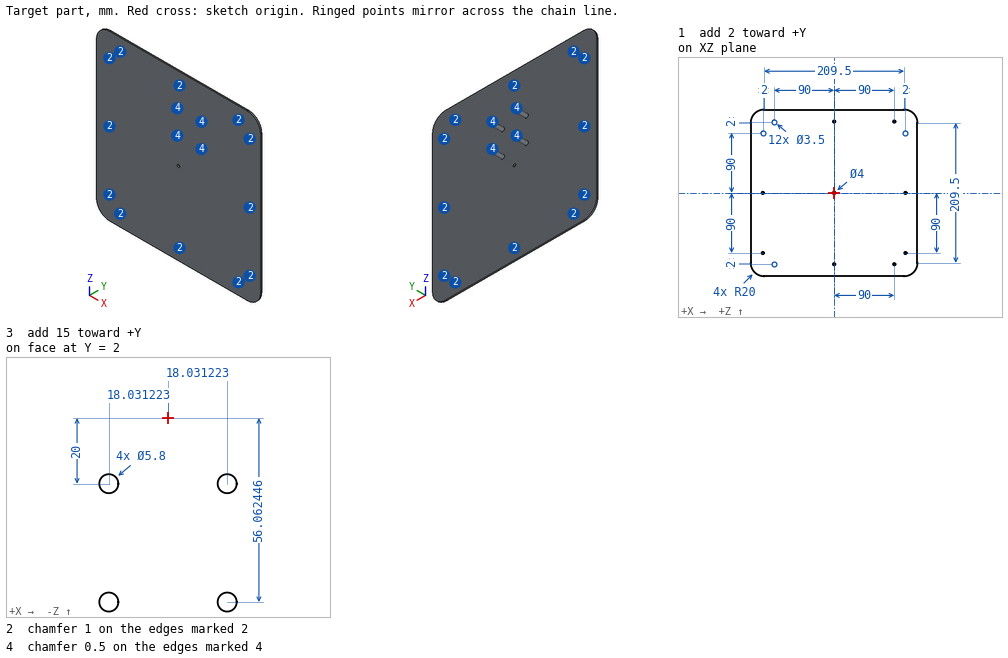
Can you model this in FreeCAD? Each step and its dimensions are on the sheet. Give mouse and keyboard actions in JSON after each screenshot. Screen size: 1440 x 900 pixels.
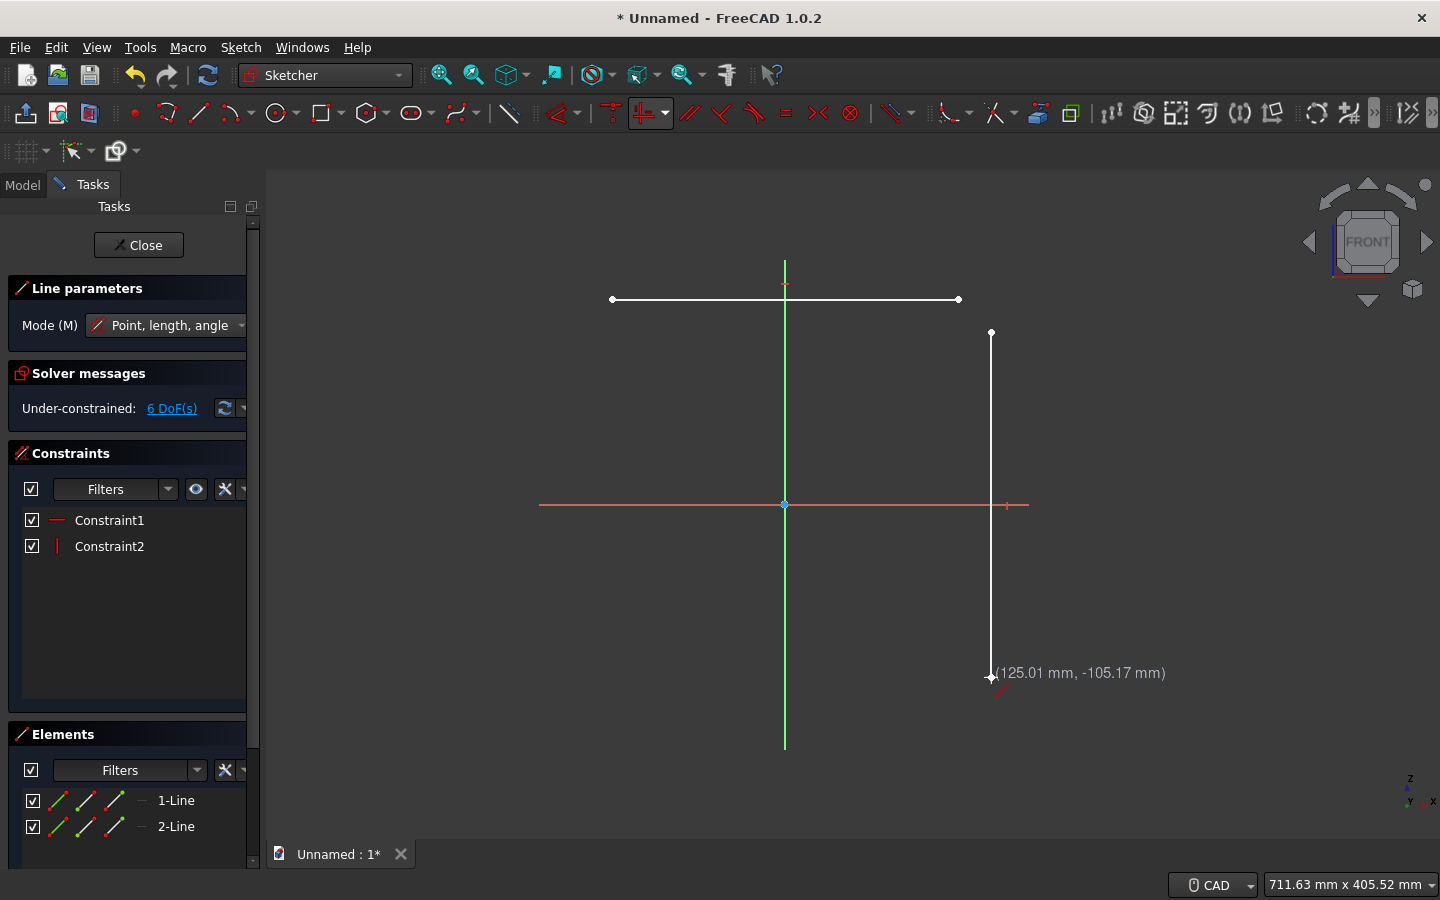
{"action": "left_click", "coordinate": [958, 710]}
{"action": "left_click", "coordinate": [612, 710]}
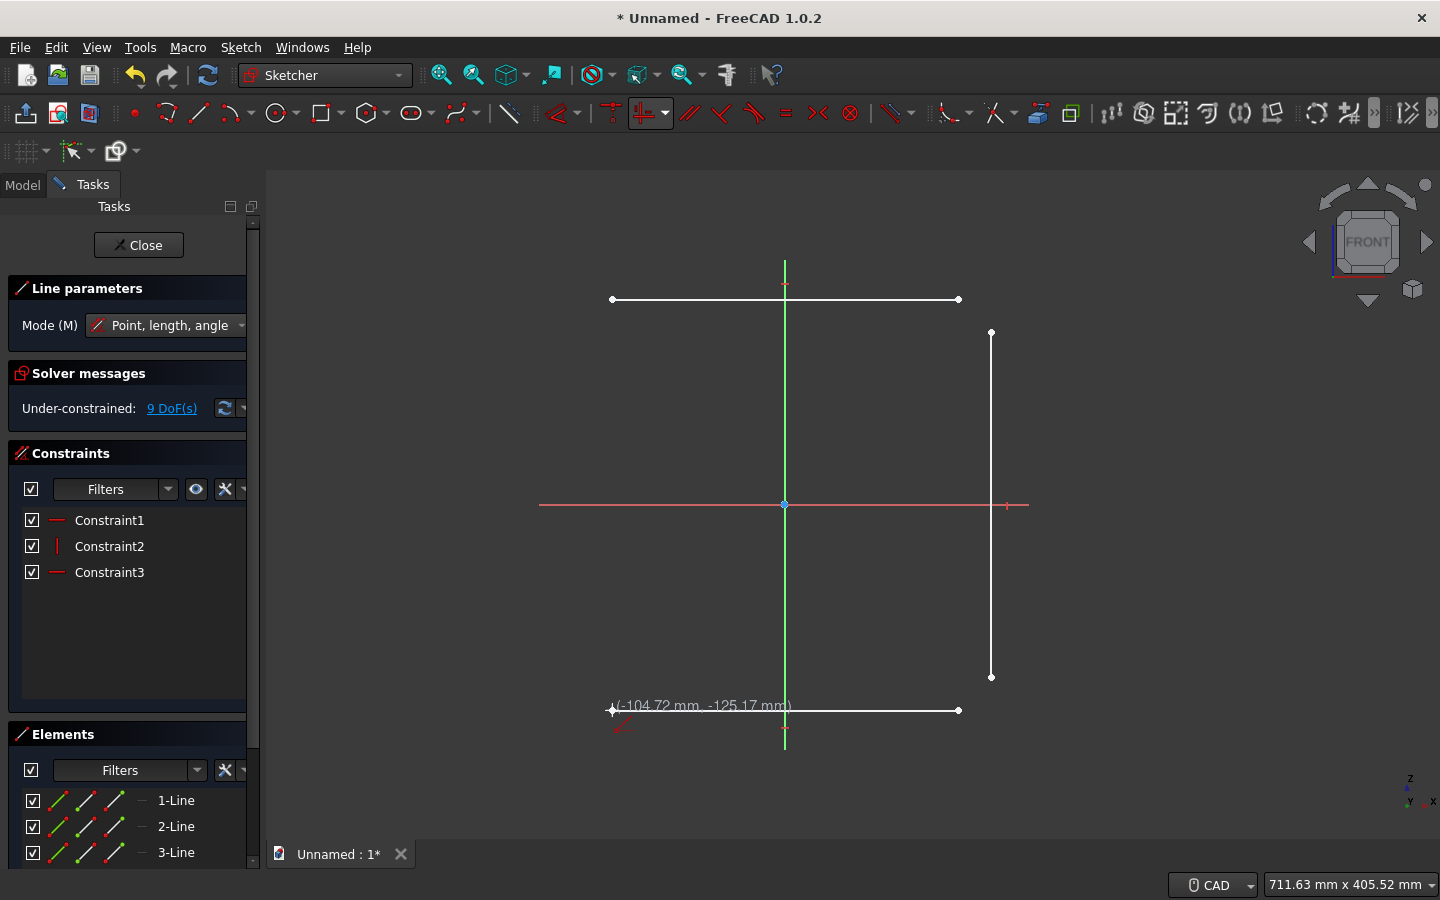
{"action": "left_click", "coordinate": [579, 677]}
{"action": "left_click", "coordinate": [579, 332]}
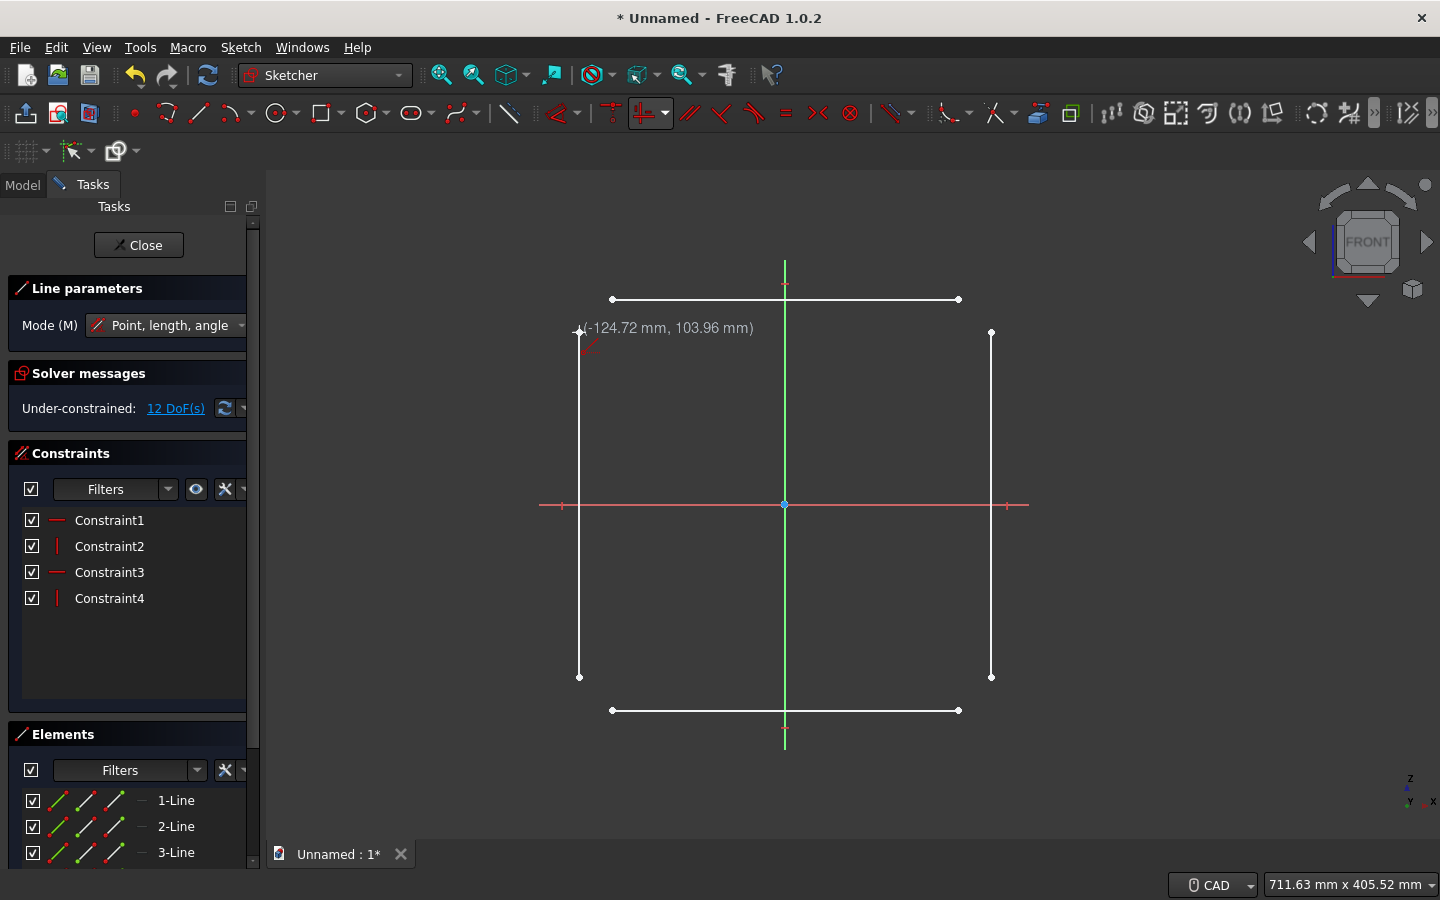
{"action": "left_click", "coordinate": [254, 114]}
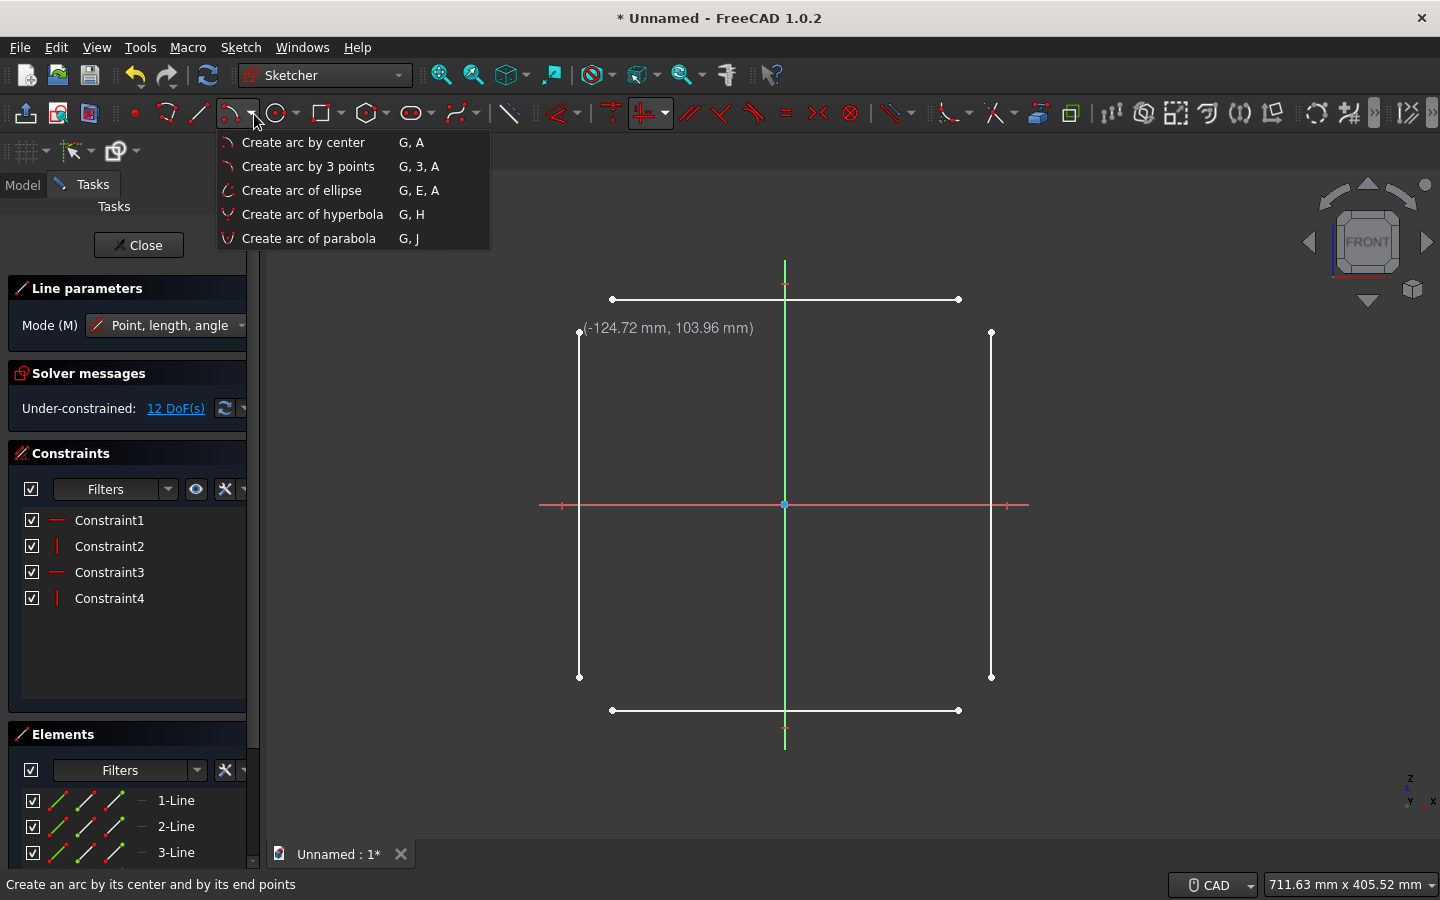
{"action": "left_click", "coordinate": [354, 166]}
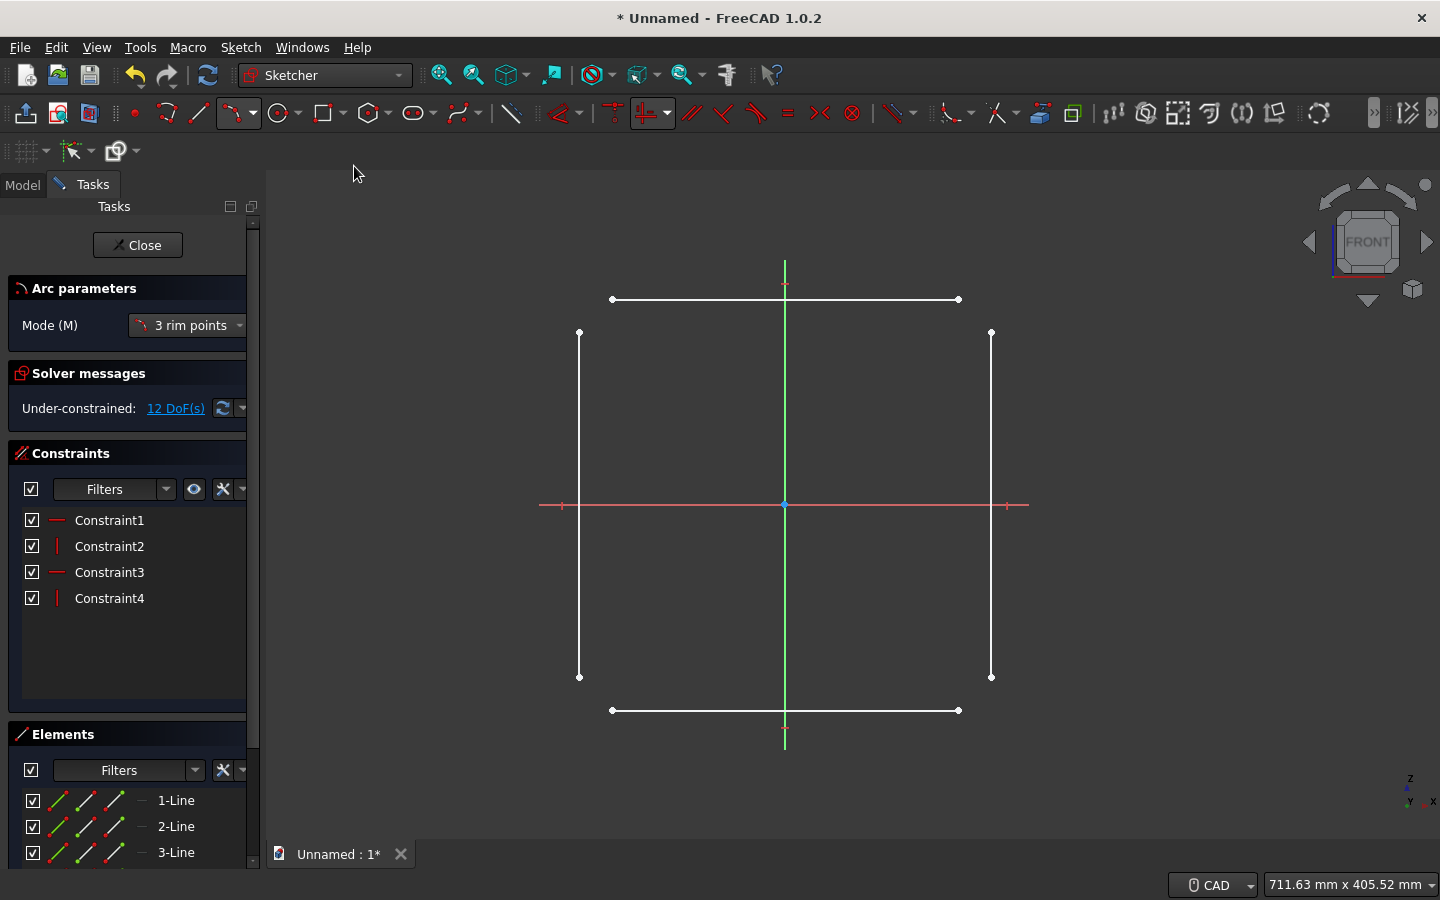
{"action": "left_click", "coordinate": [958, 300]}
{"action": "left_click", "coordinate": [991, 333]}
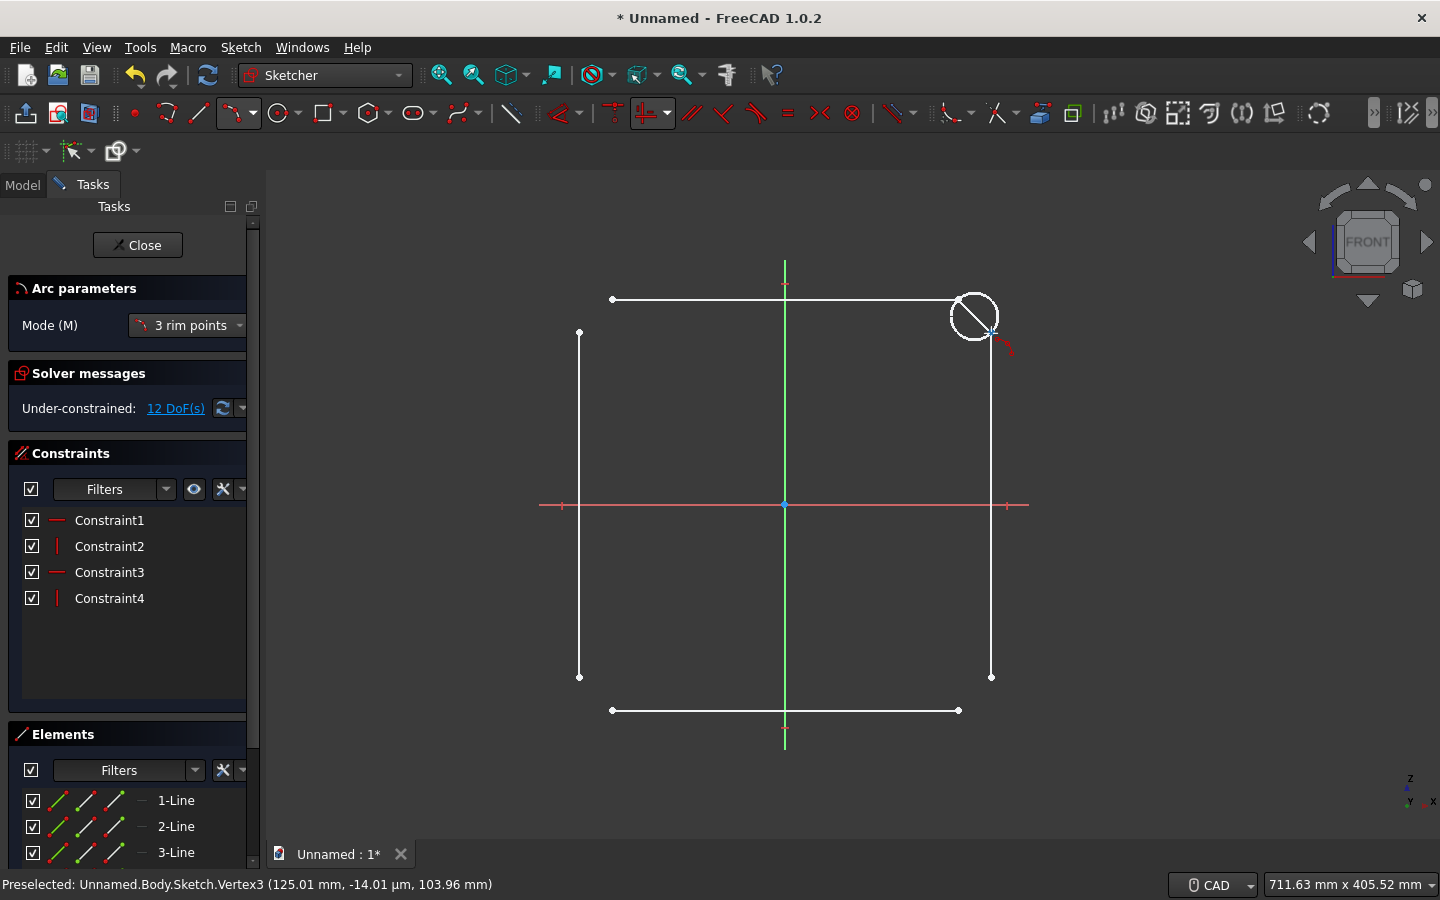
{"action": "scroll", "coordinate": [981, 308], "scroll_direction": "up", "scroll_amount": 3}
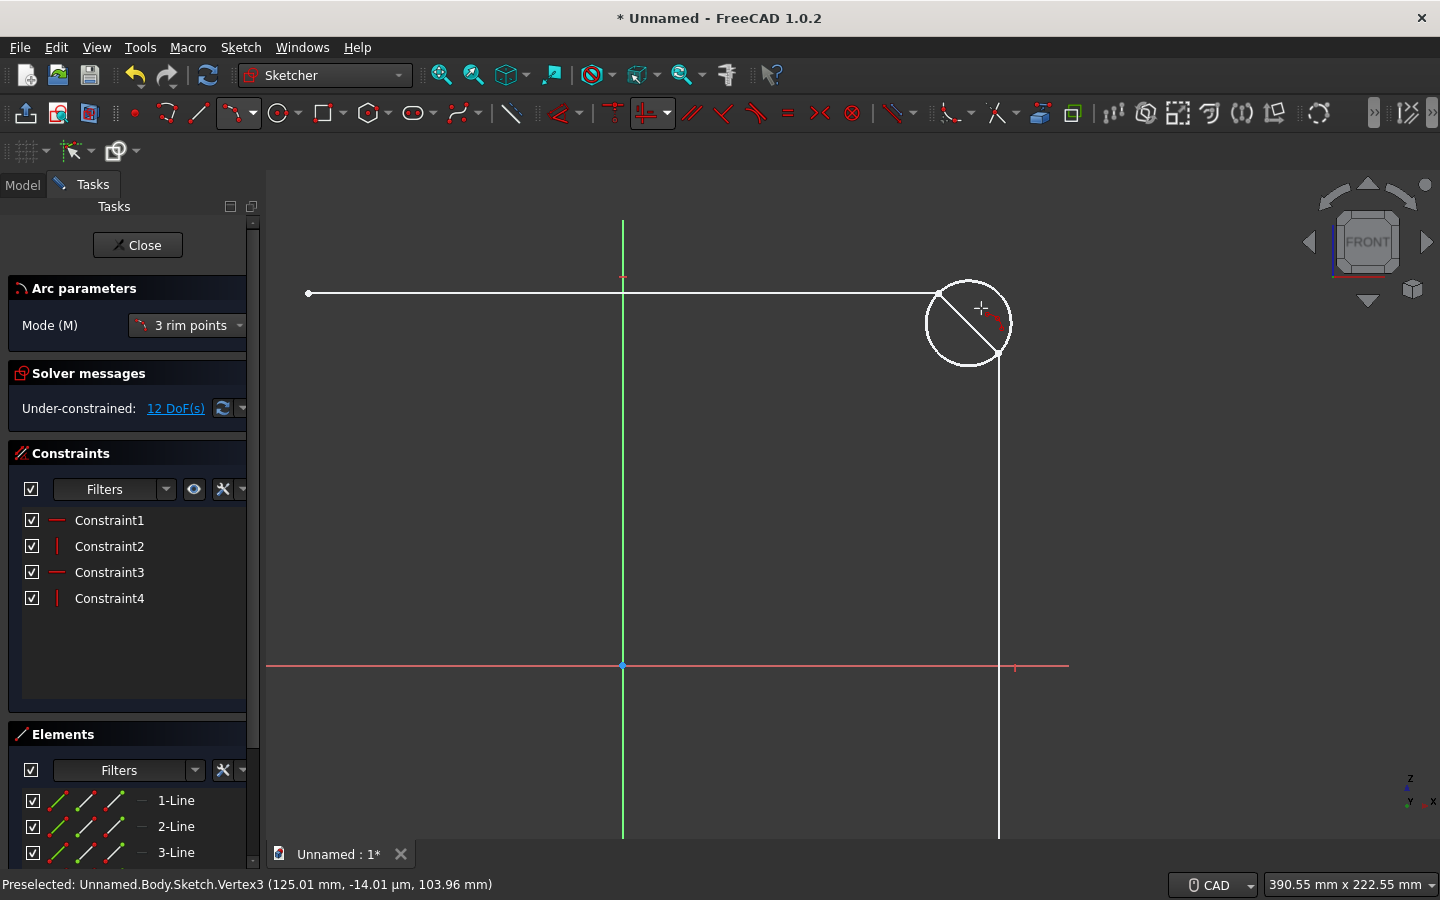
{"action": "left_click", "coordinate": [980, 308]}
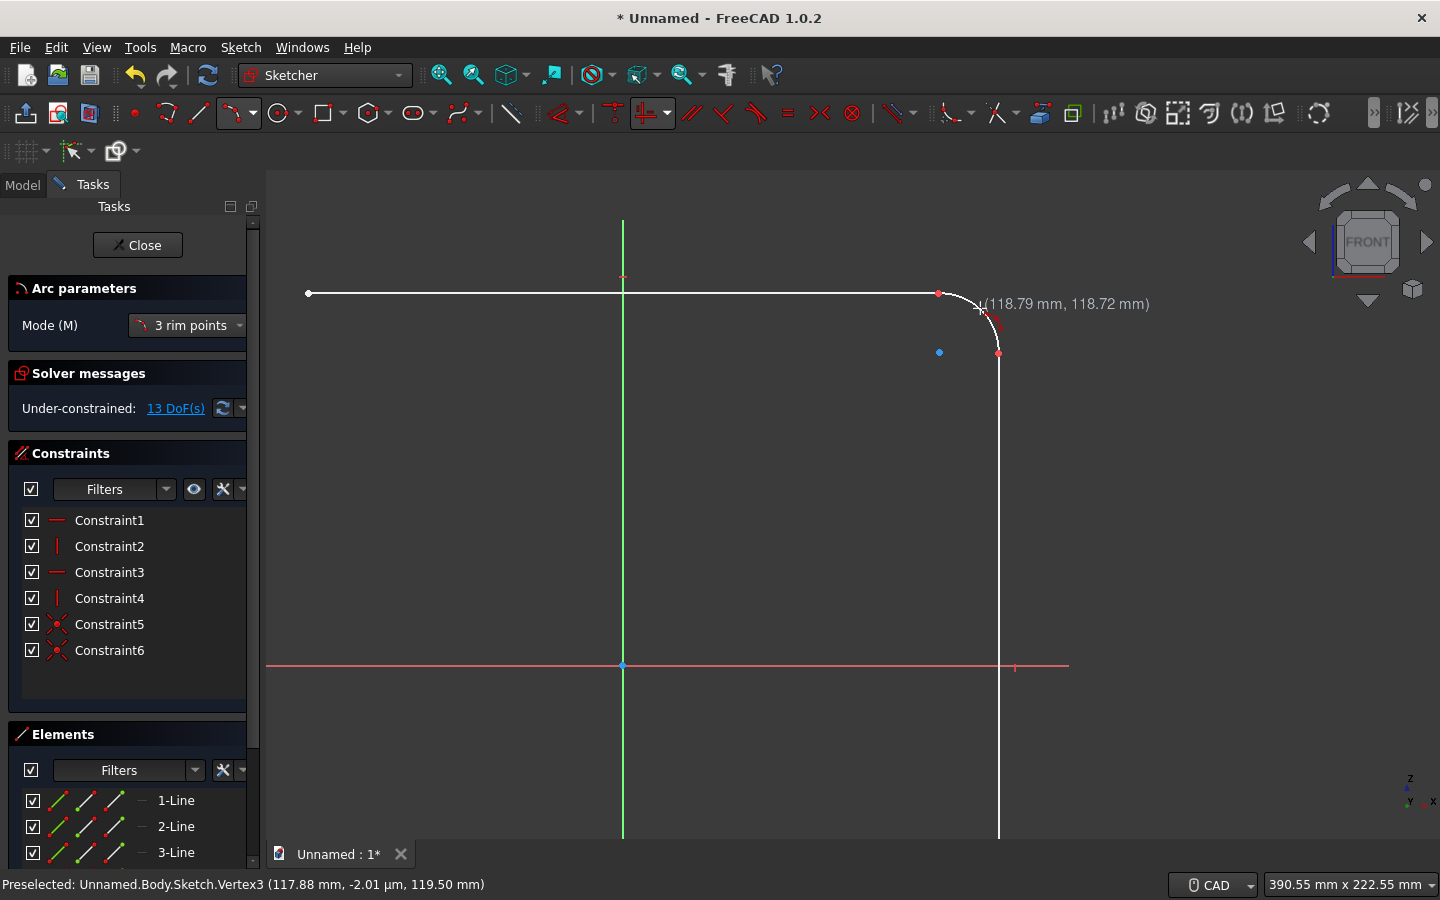
{"action": "scroll", "coordinate": [981, 308], "scroll_direction": "down", "scroll_amount": 3}